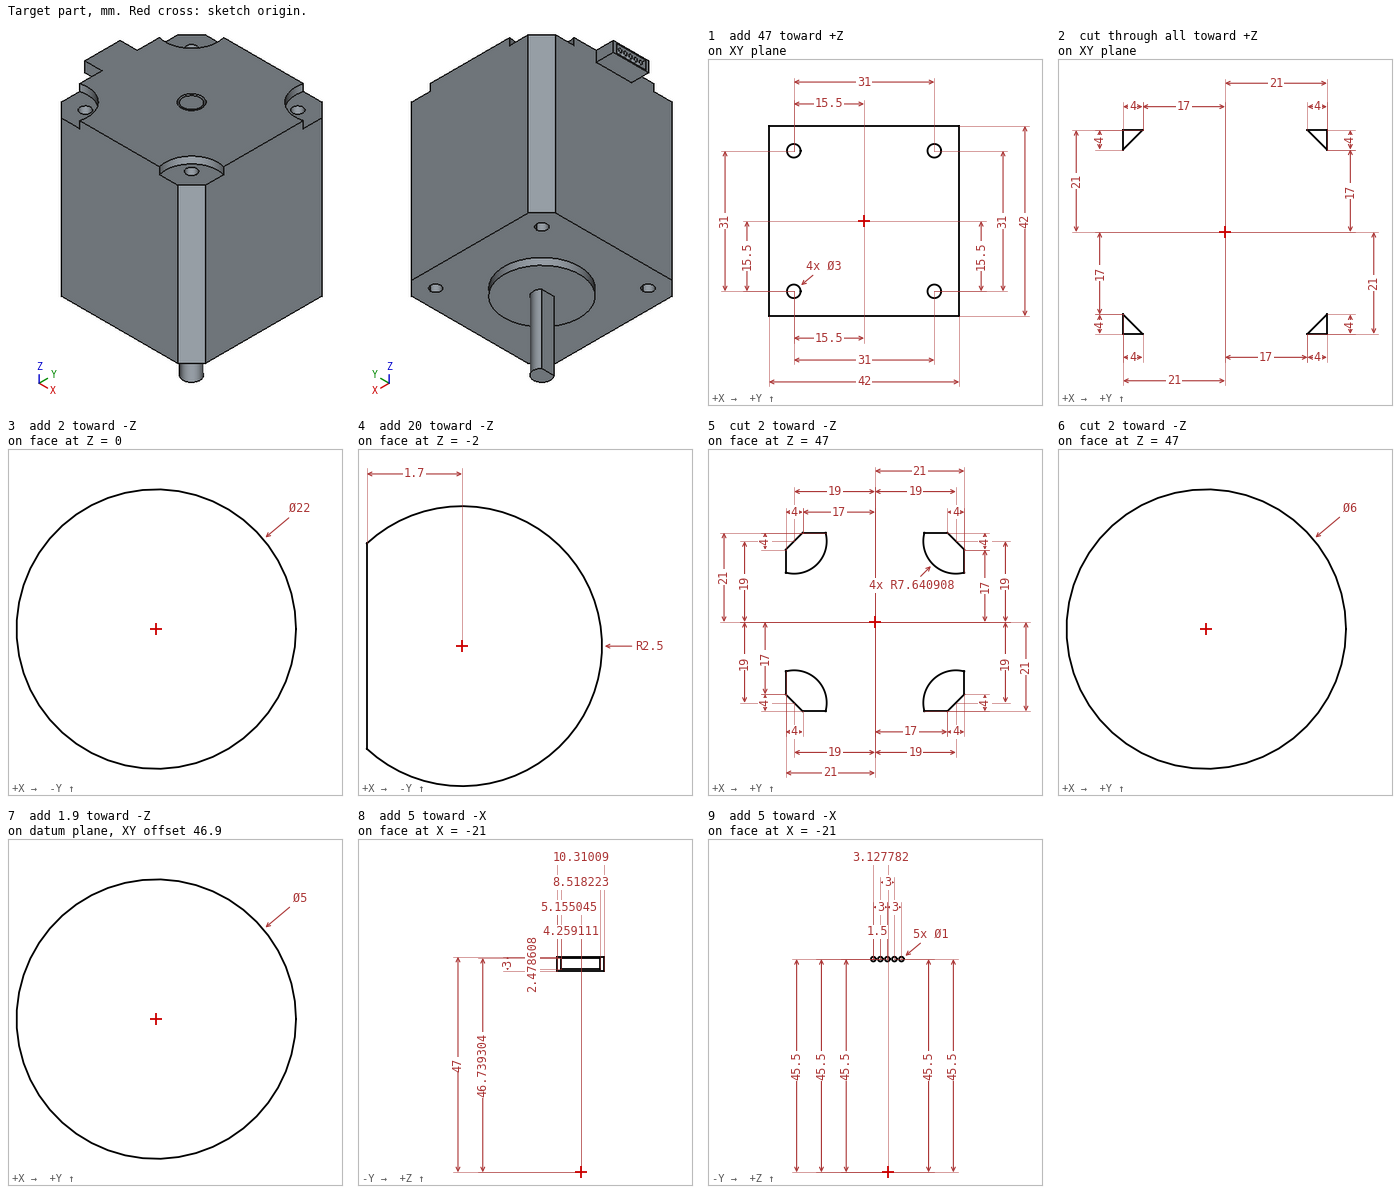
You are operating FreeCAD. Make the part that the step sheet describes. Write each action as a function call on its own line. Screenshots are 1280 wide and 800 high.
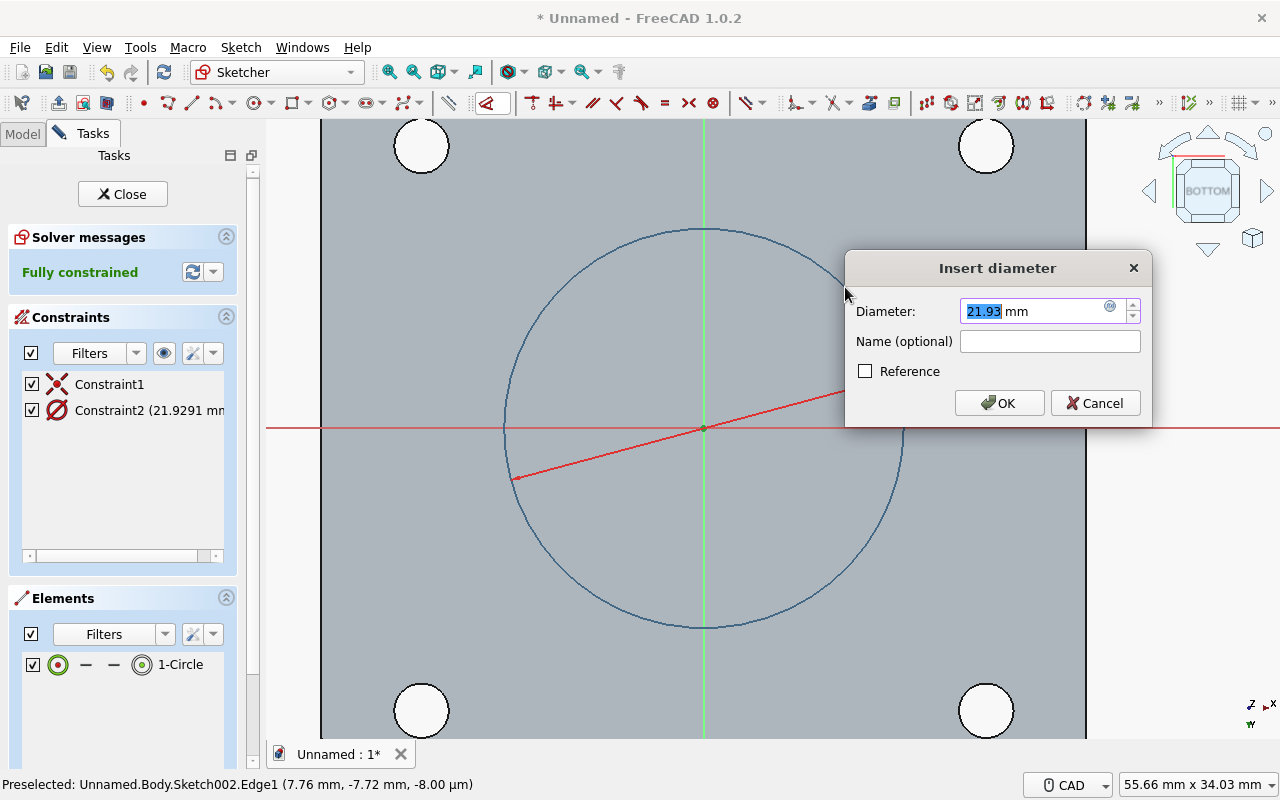
text(22)
key(Return)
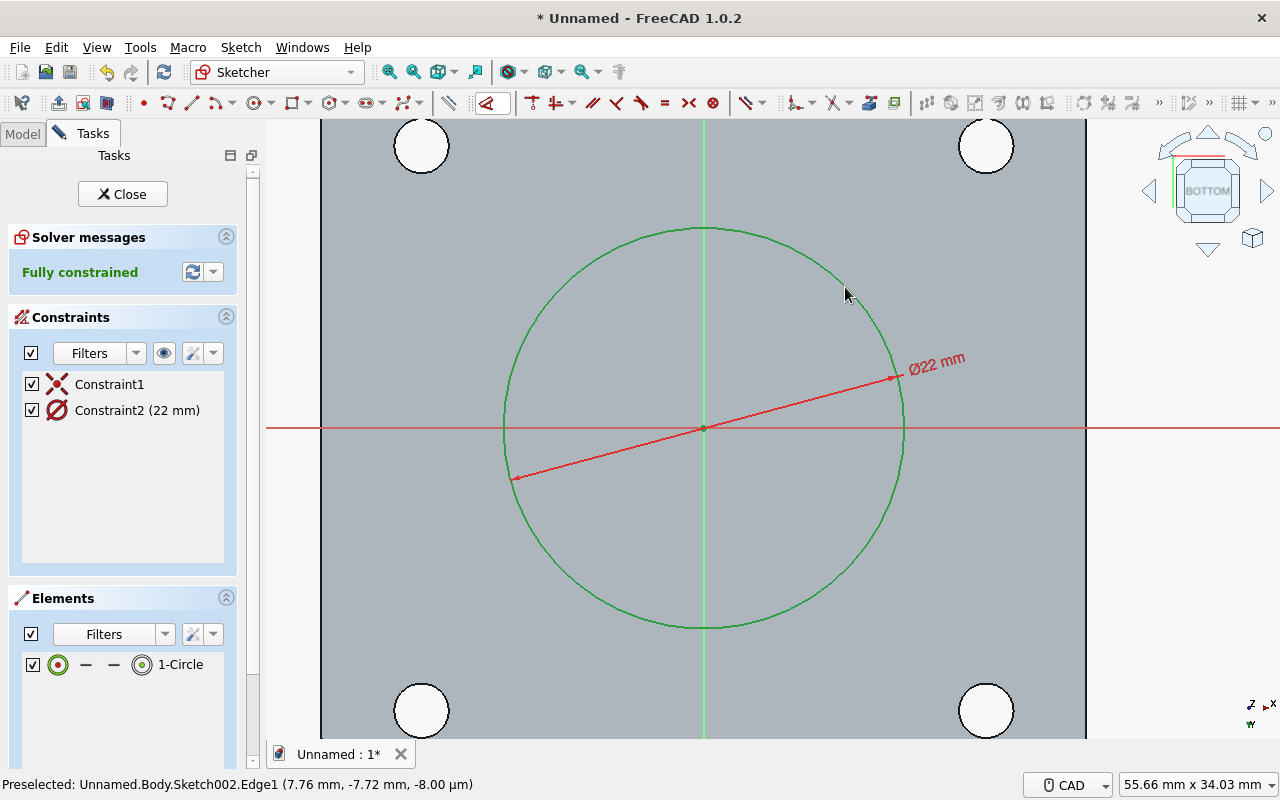
click(123, 194)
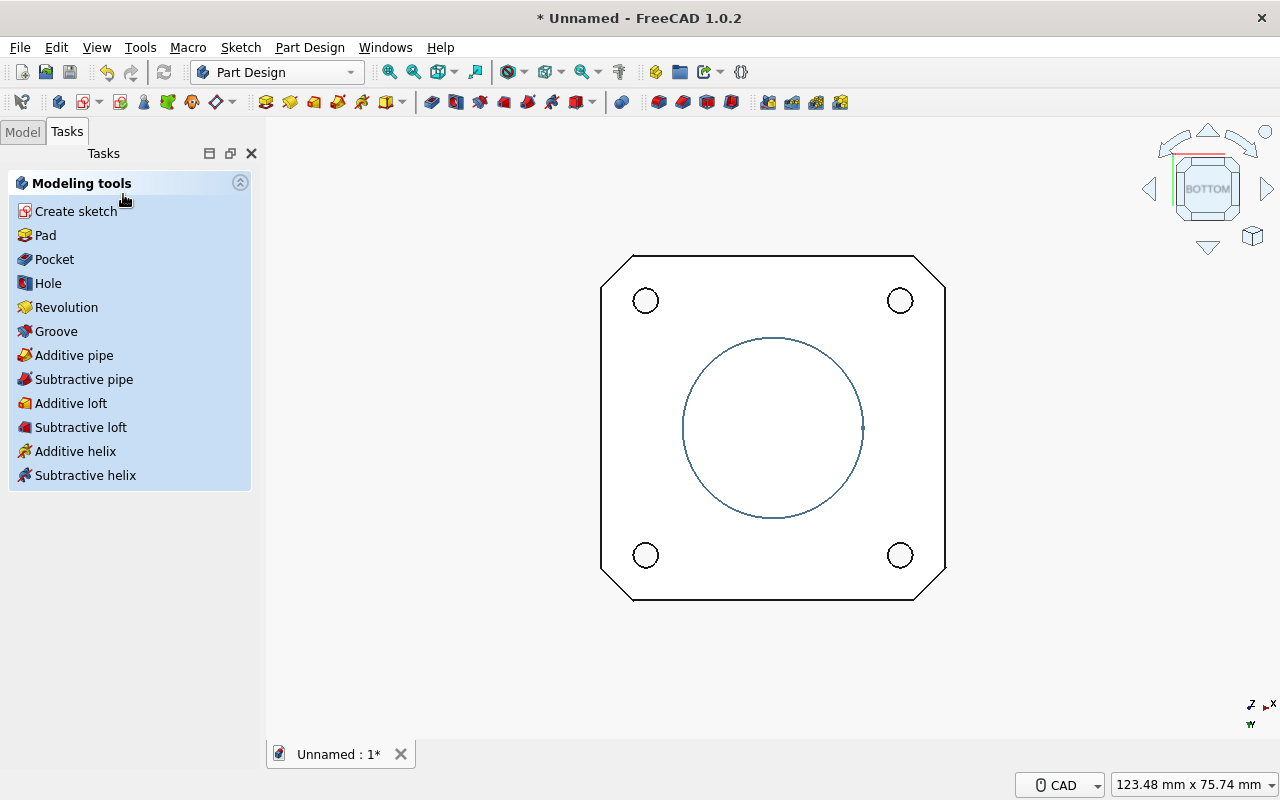
click(266, 102)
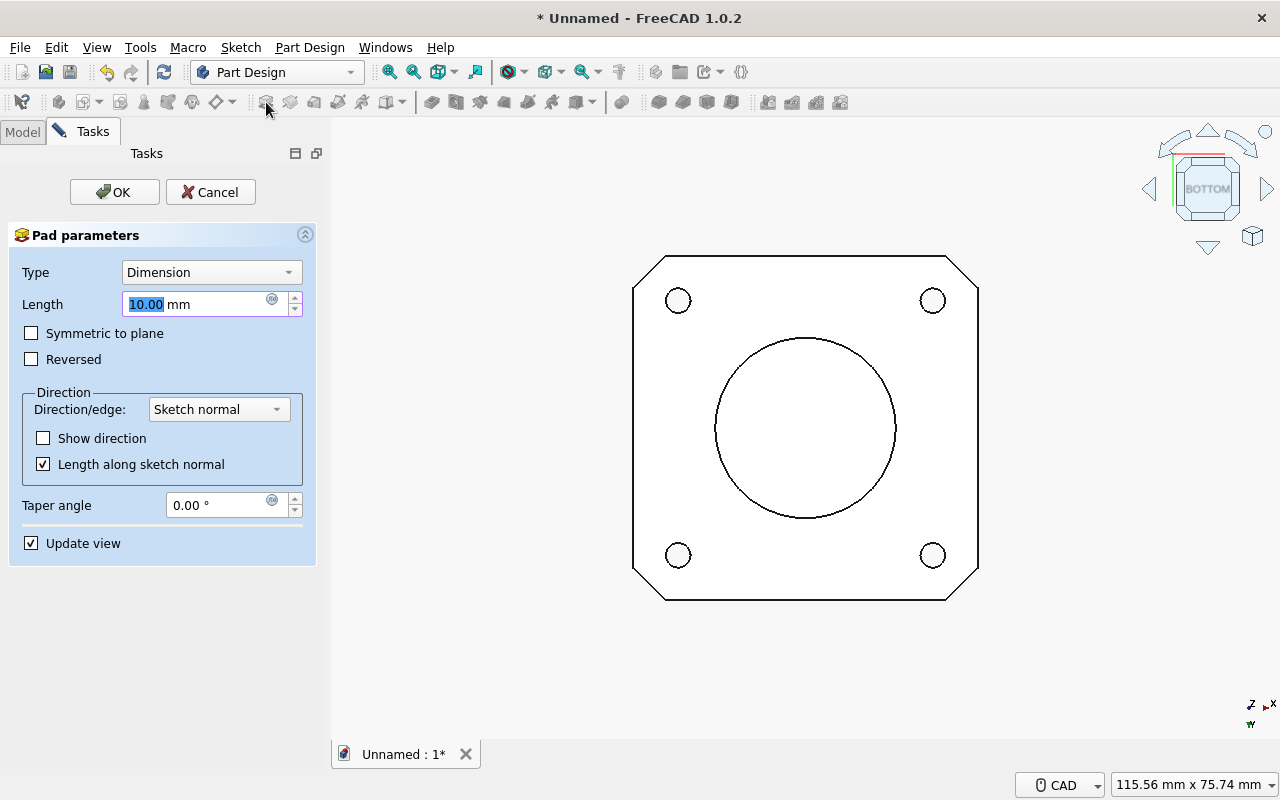
text(2)
key(Tab)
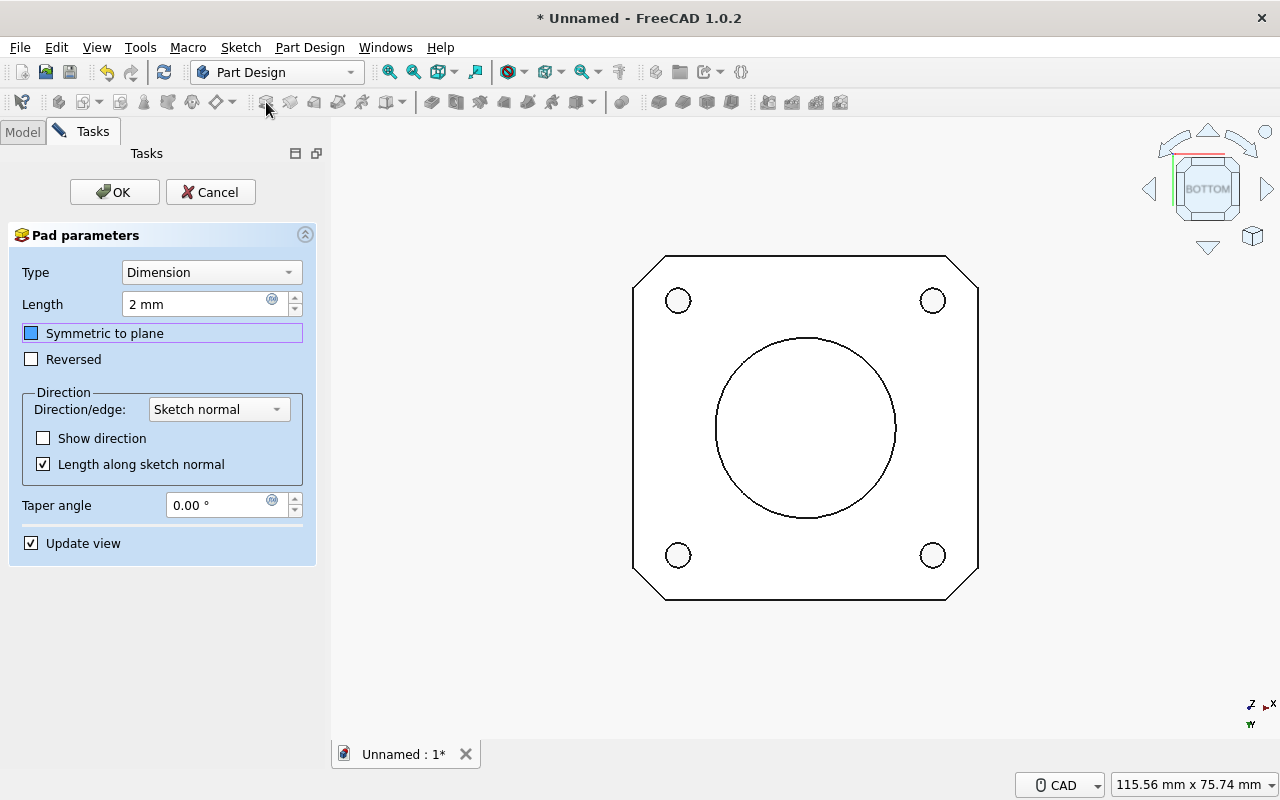
click(115, 192)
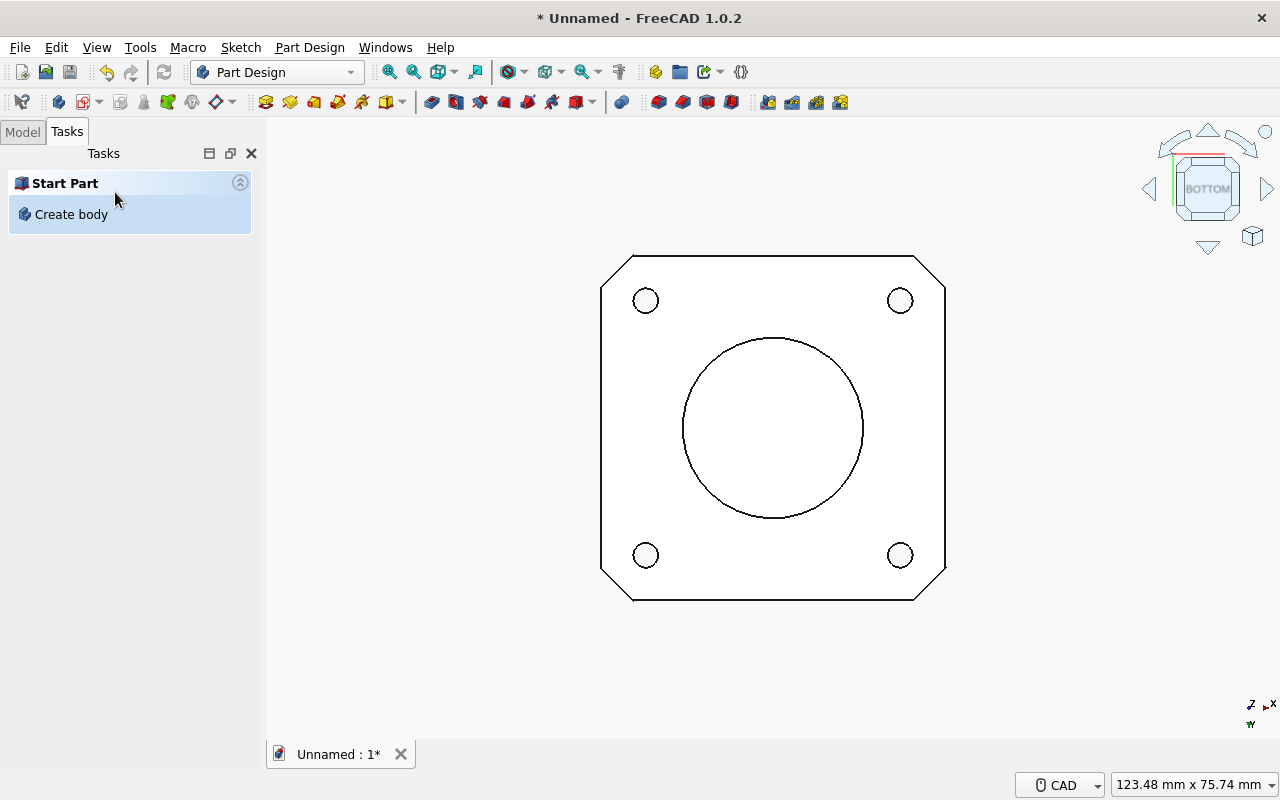
click(773, 427)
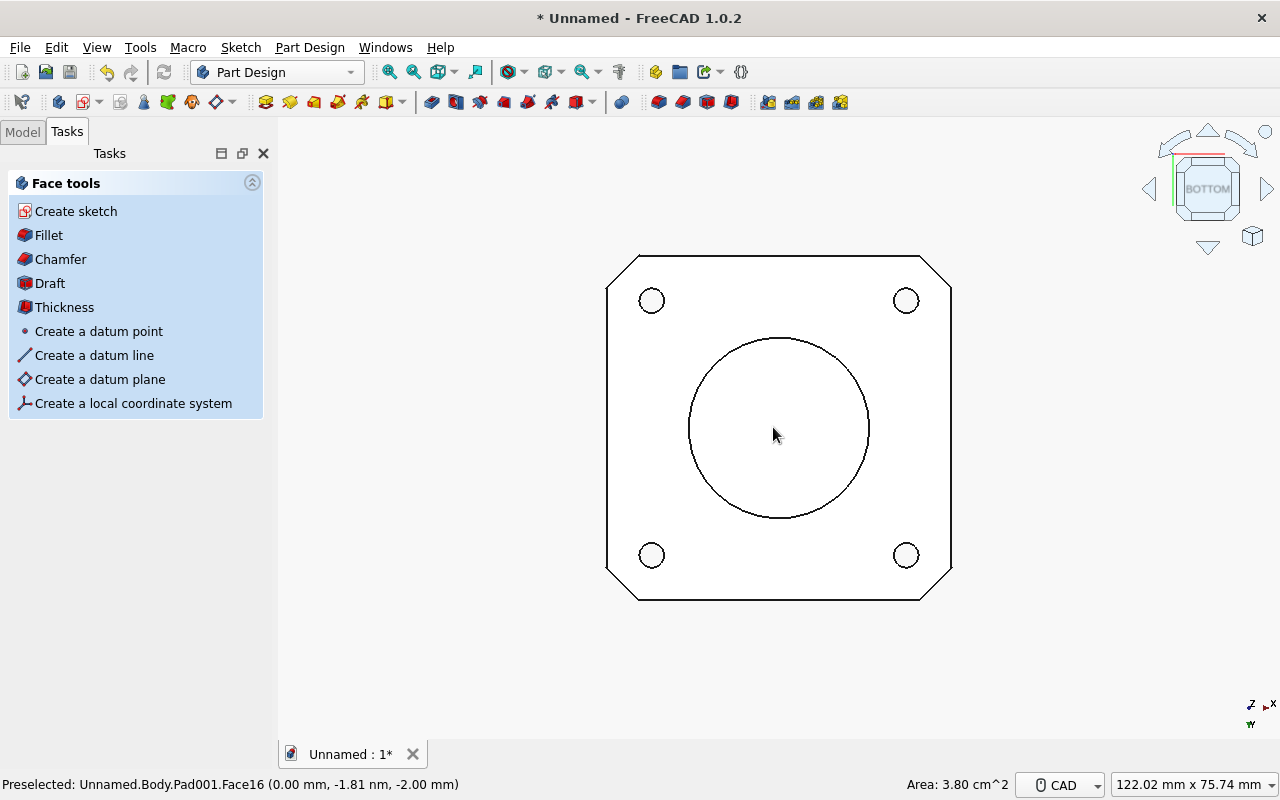
click(84, 102)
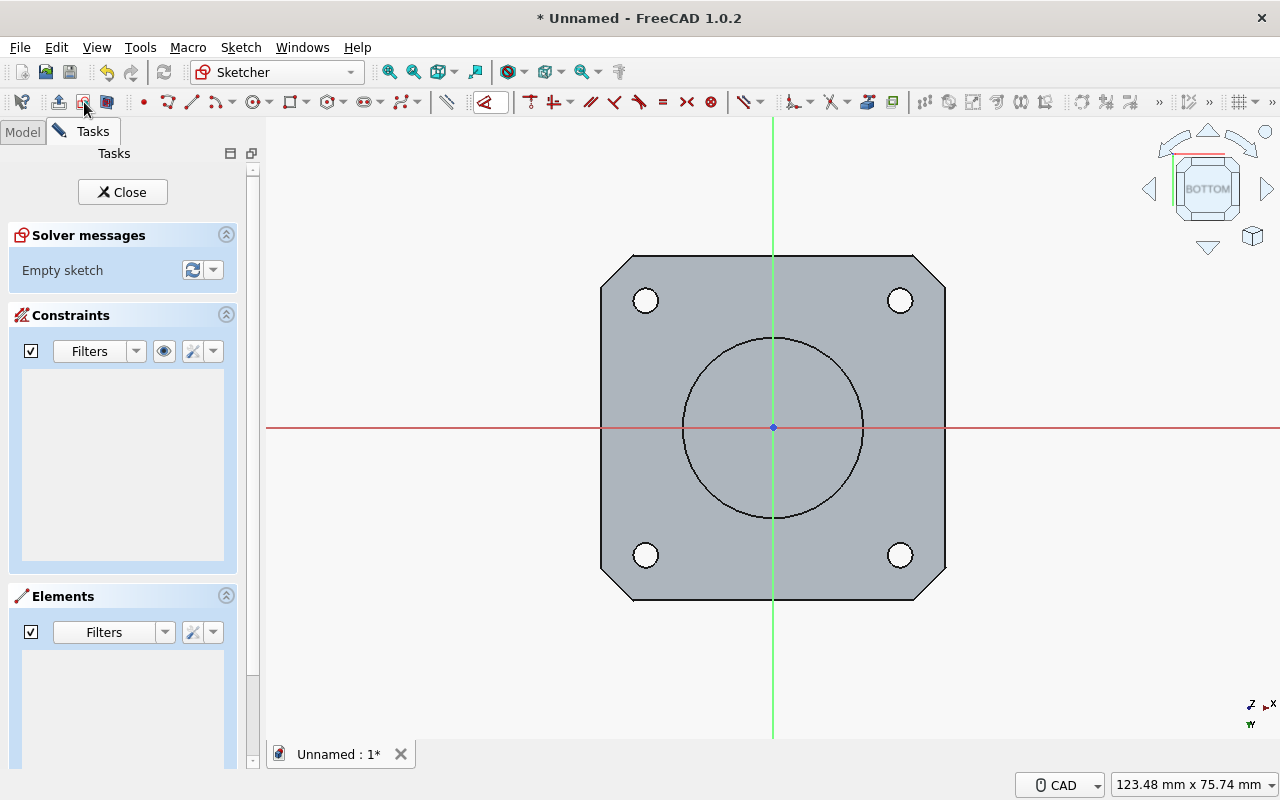
scroll(782, 428, up, 13)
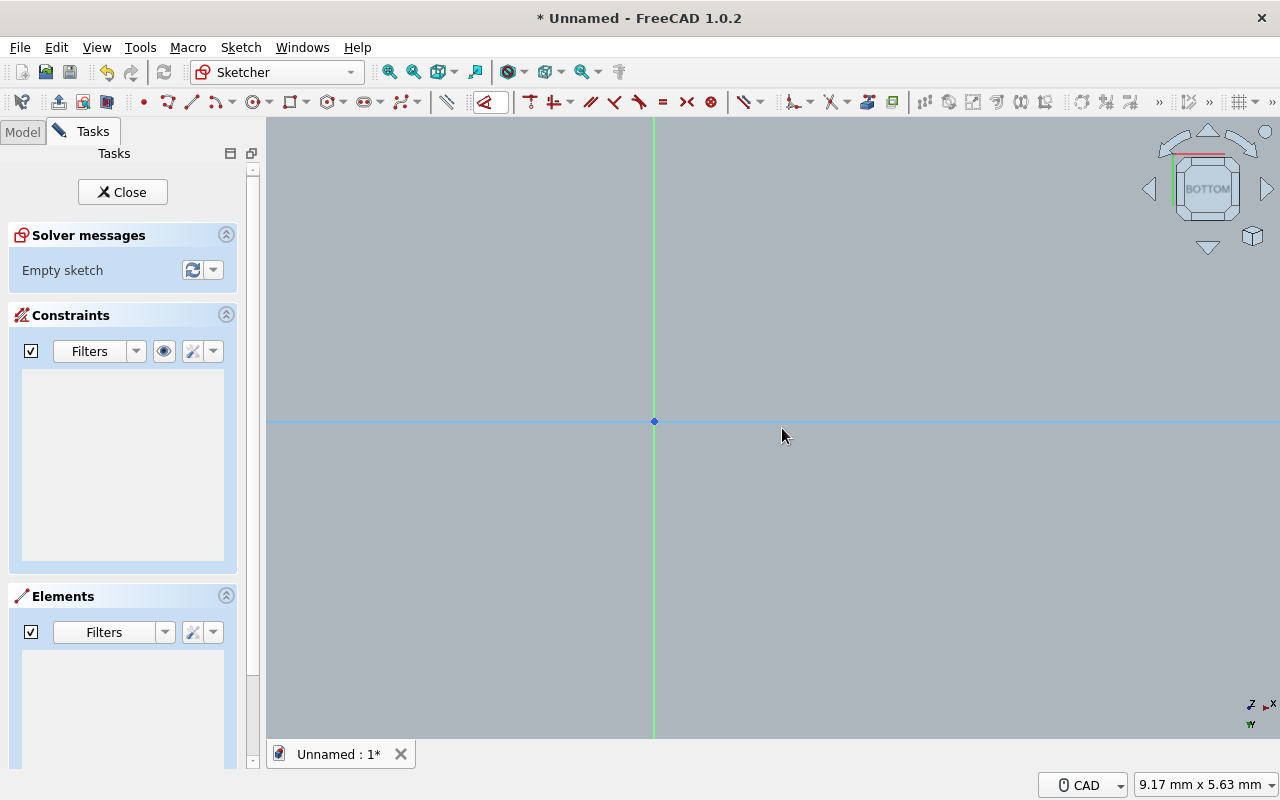
key(g)
key(l)